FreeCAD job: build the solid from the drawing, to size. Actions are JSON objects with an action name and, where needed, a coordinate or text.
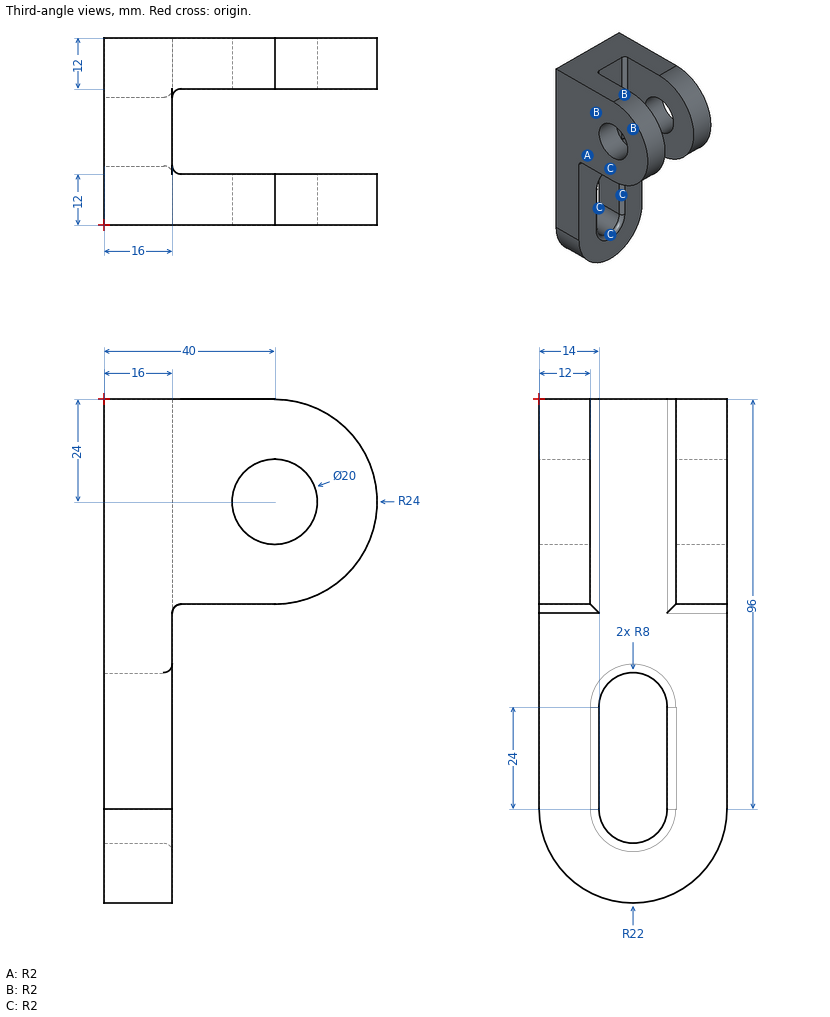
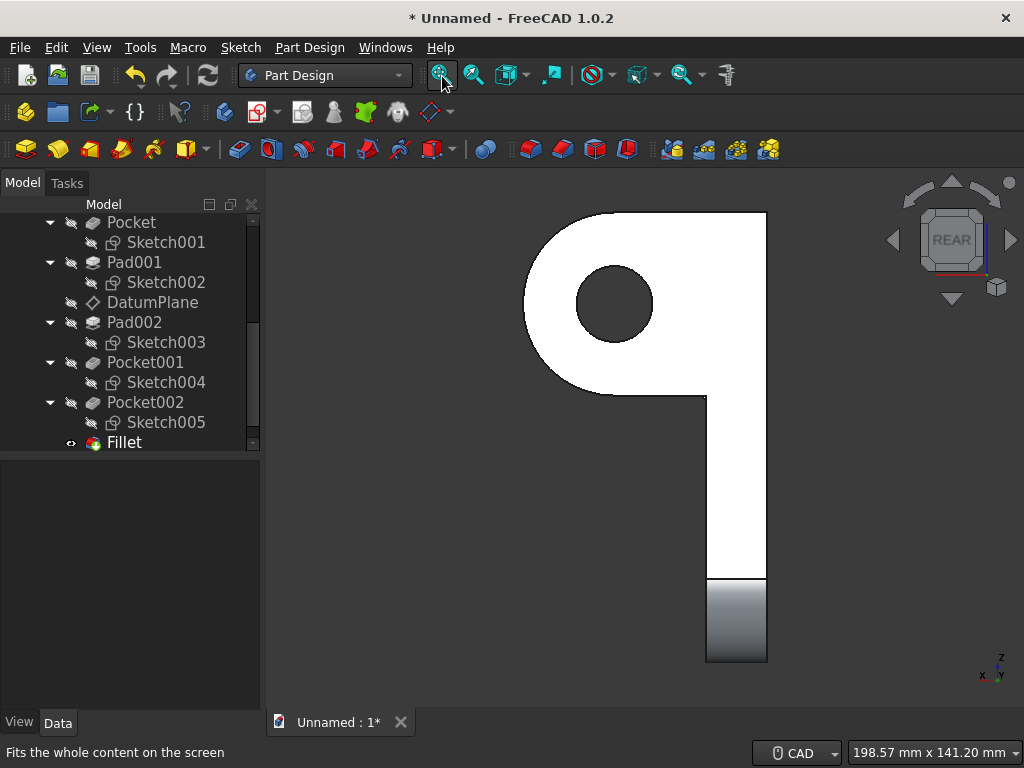
{"action": "key", "text": "6"}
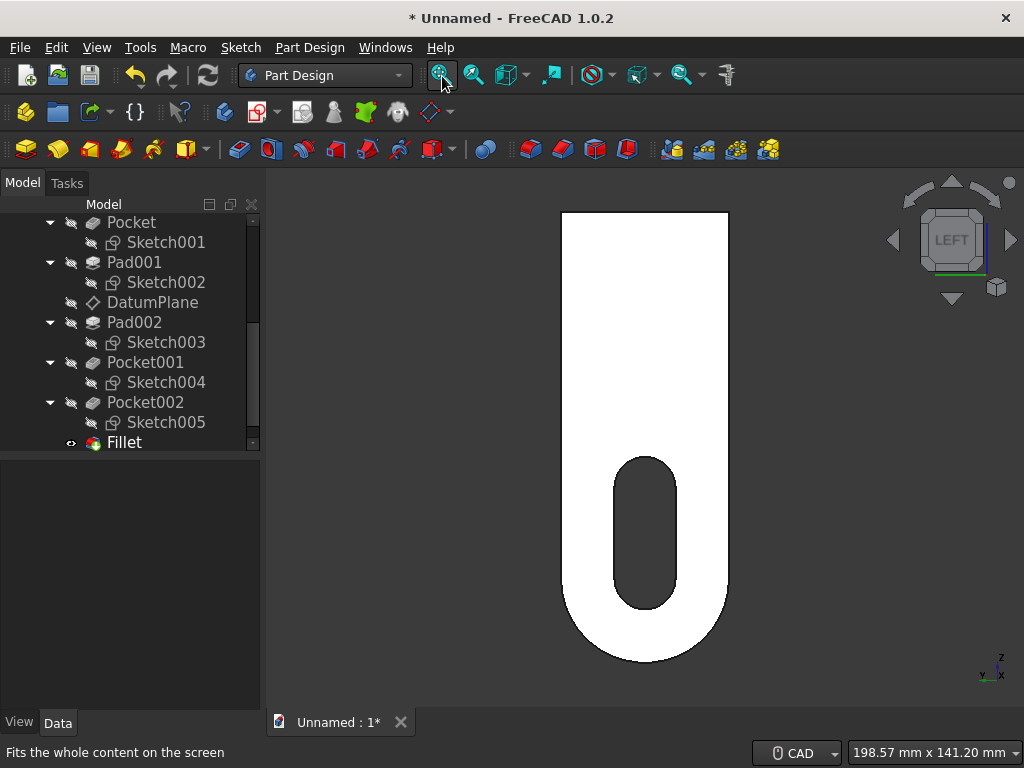
{"action": "key", "text": "v 3"}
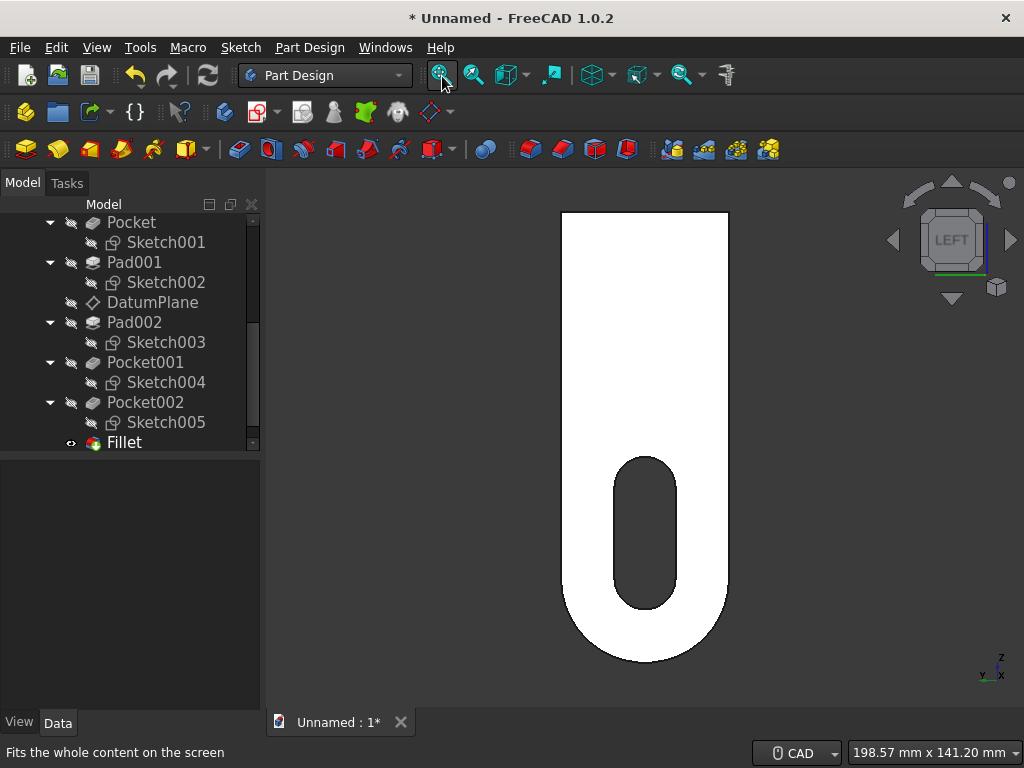
{"action": "key", "text": "0"}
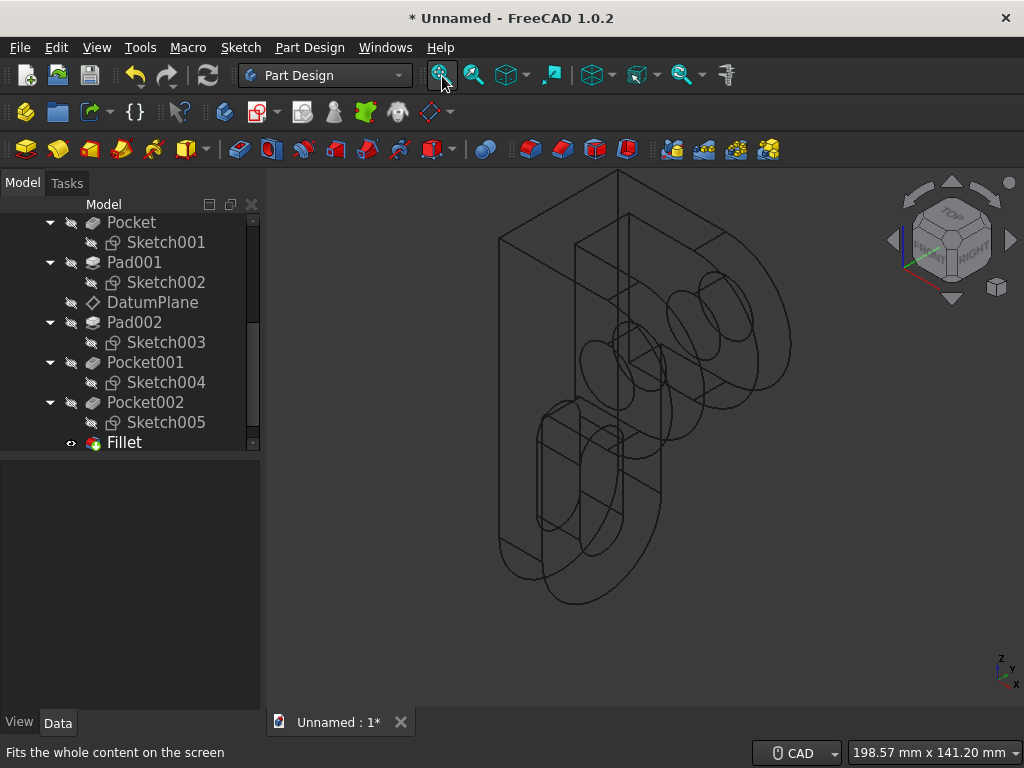
{"action": "left_click", "coordinate": [575, 318]}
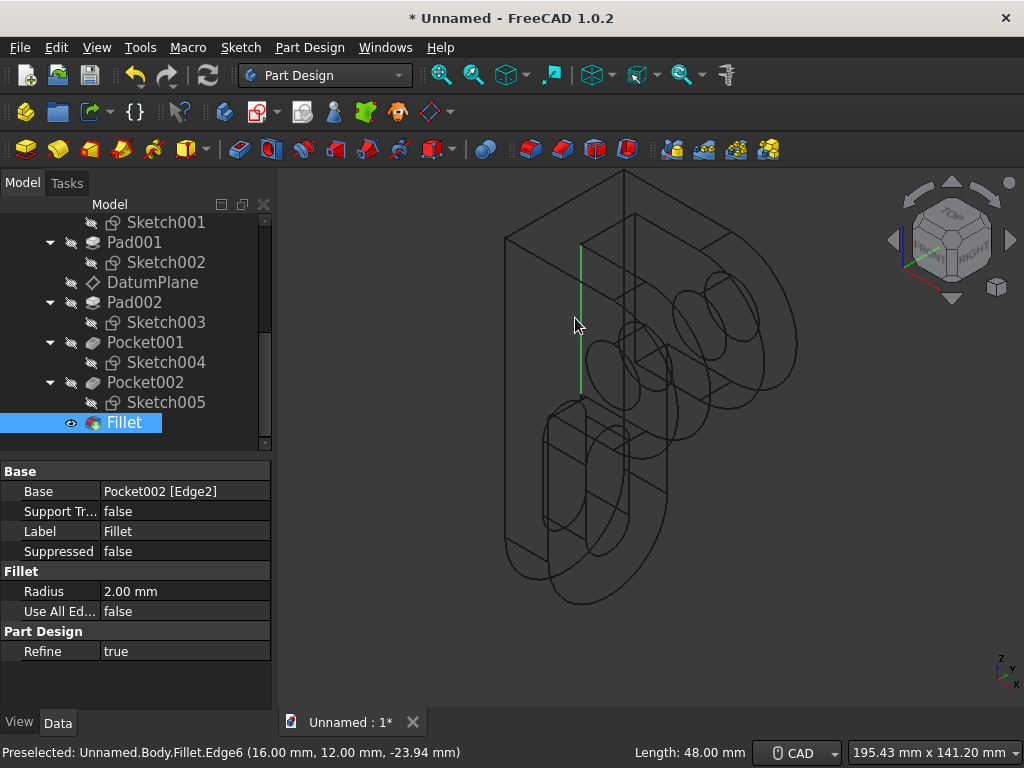
{"action": "left_click", "coordinate": [635, 302], "text": "ctrl"}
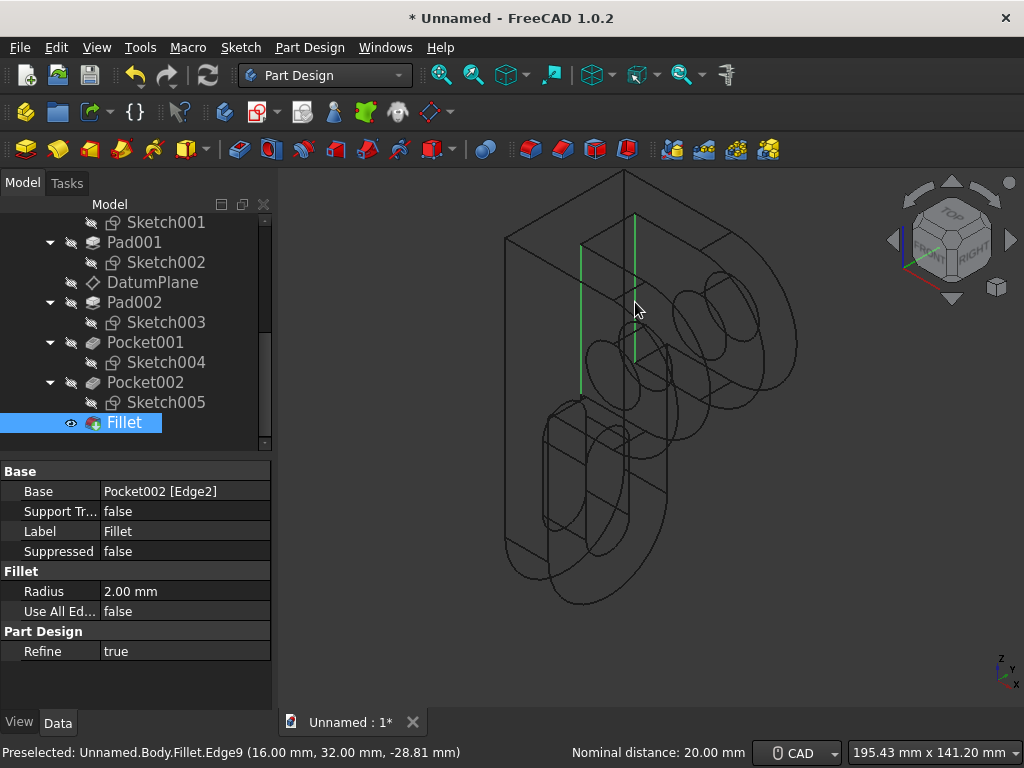
{"action": "left_click", "coordinate": [651, 352], "text": "ctrl"}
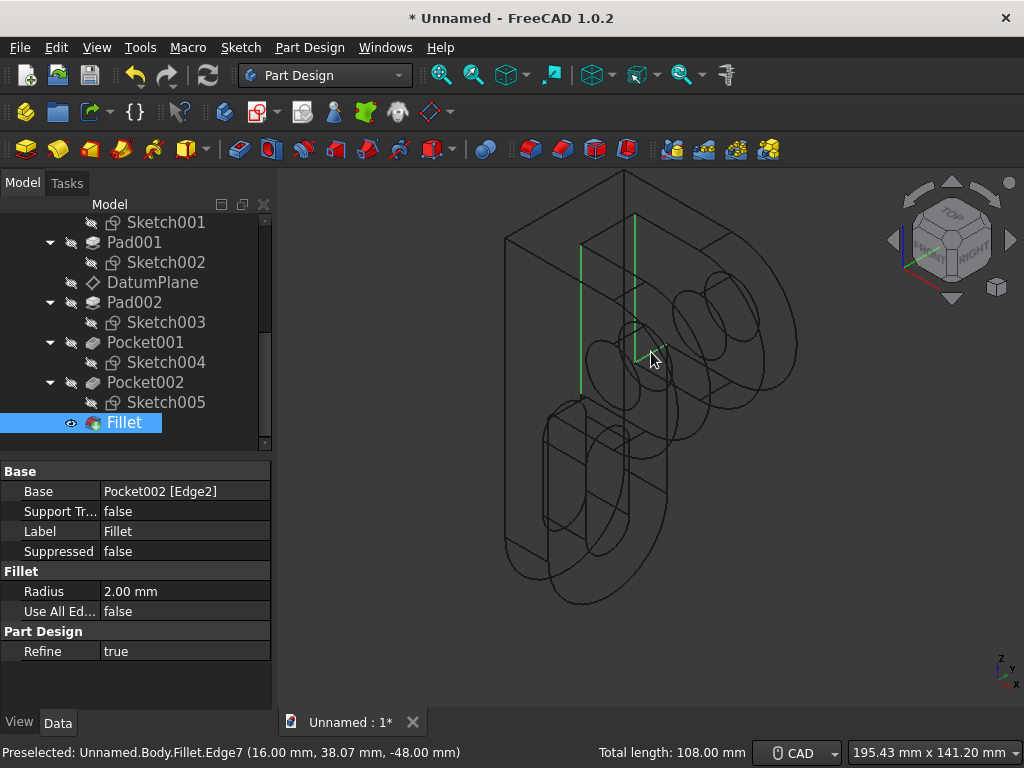
{"action": "key", "text": "v 1"}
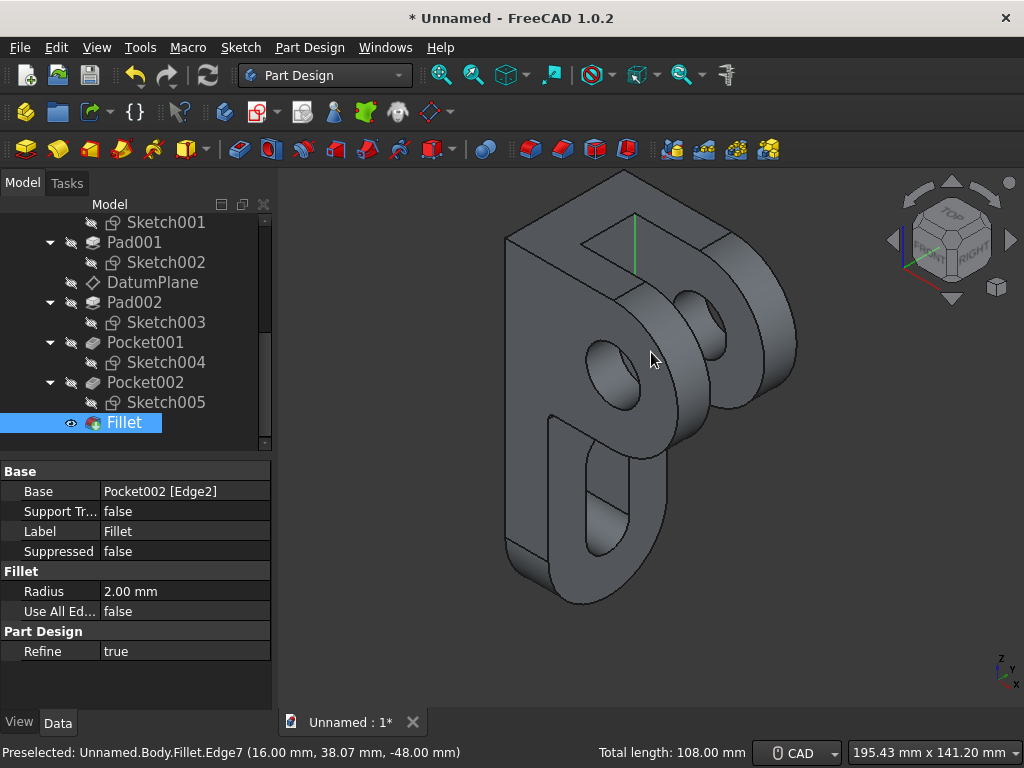
{"action": "left_click", "coordinate": [532, 150]}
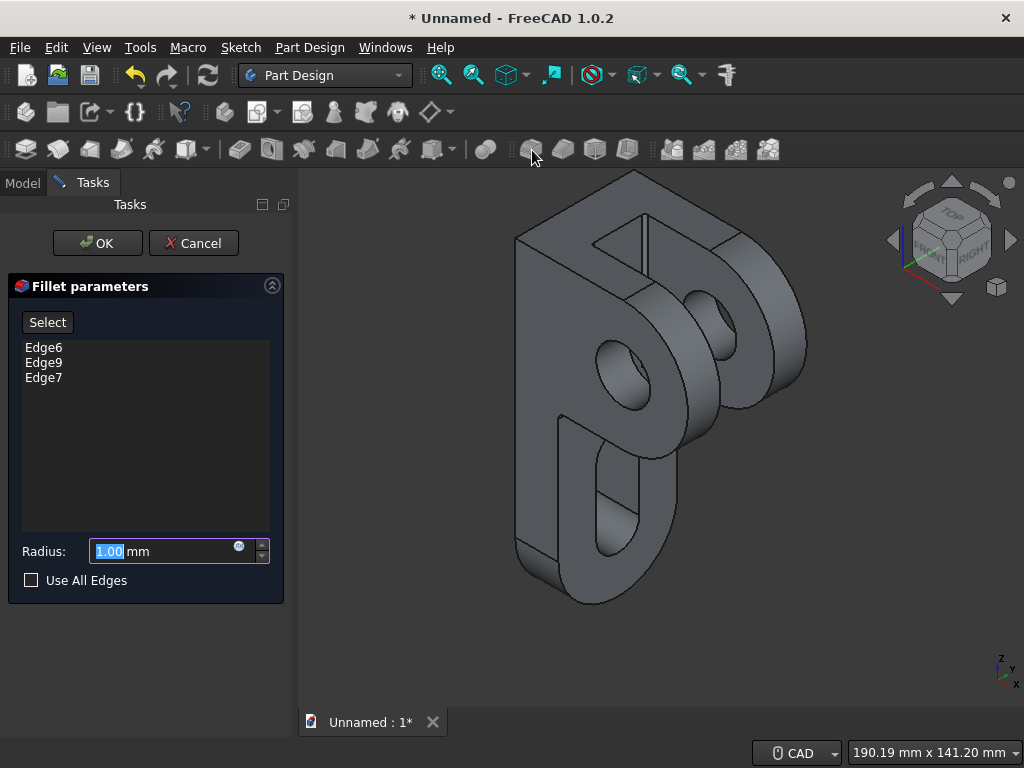
{"action": "type", "text": "2"}
{"action": "key", "text": "Tab"}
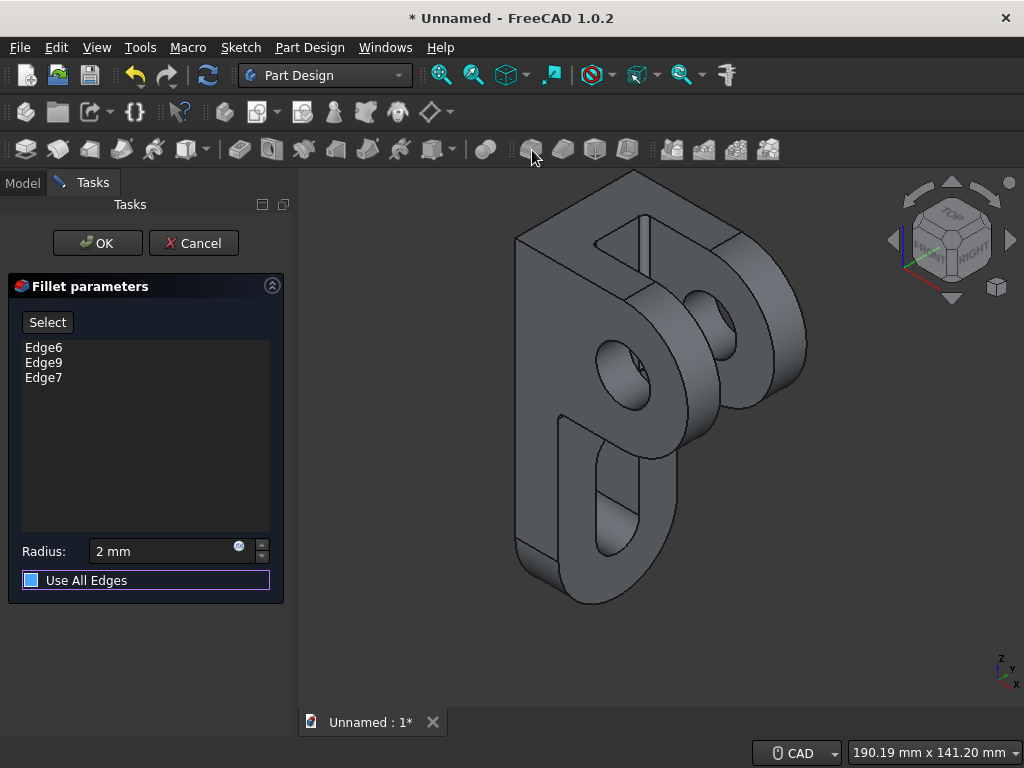
{"action": "left_click", "coordinate": [98, 243]}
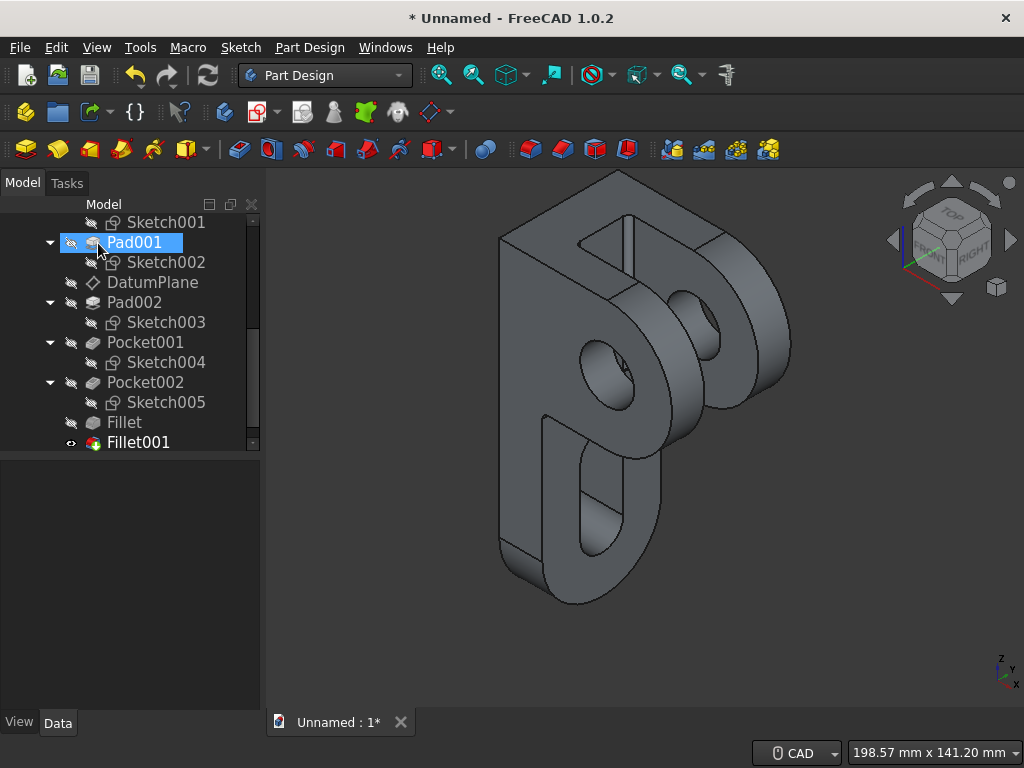
{"action": "left_click", "coordinate": [602, 552]}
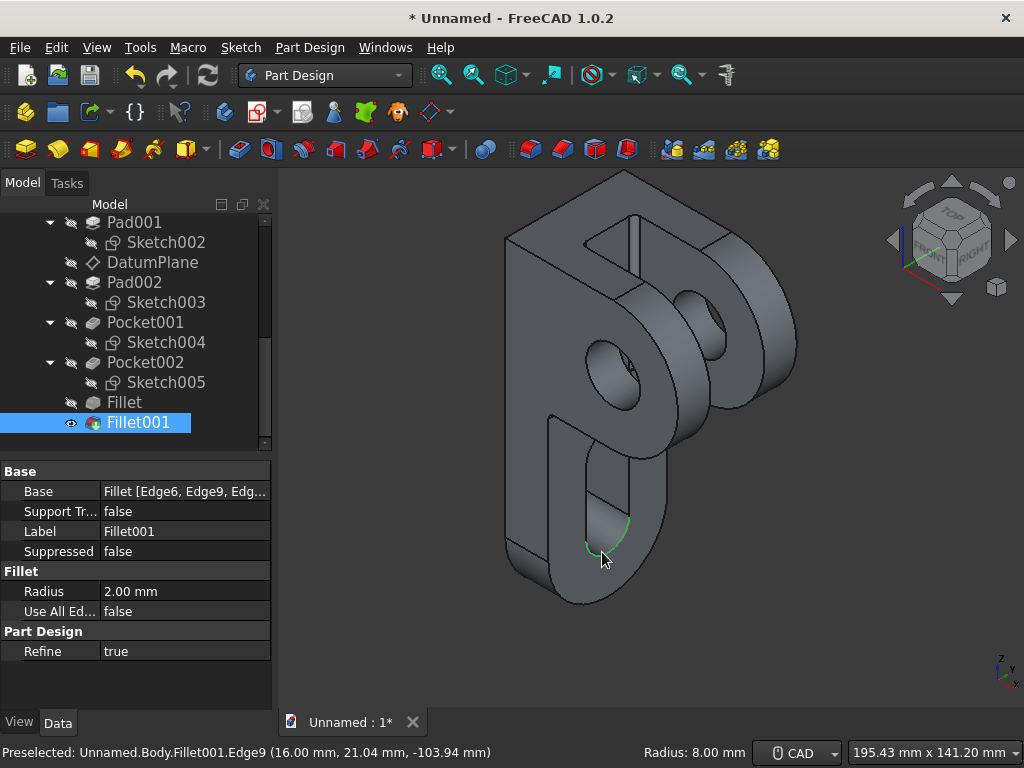
{"action": "left_click", "coordinate": [629, 477], "text": "ctrl"}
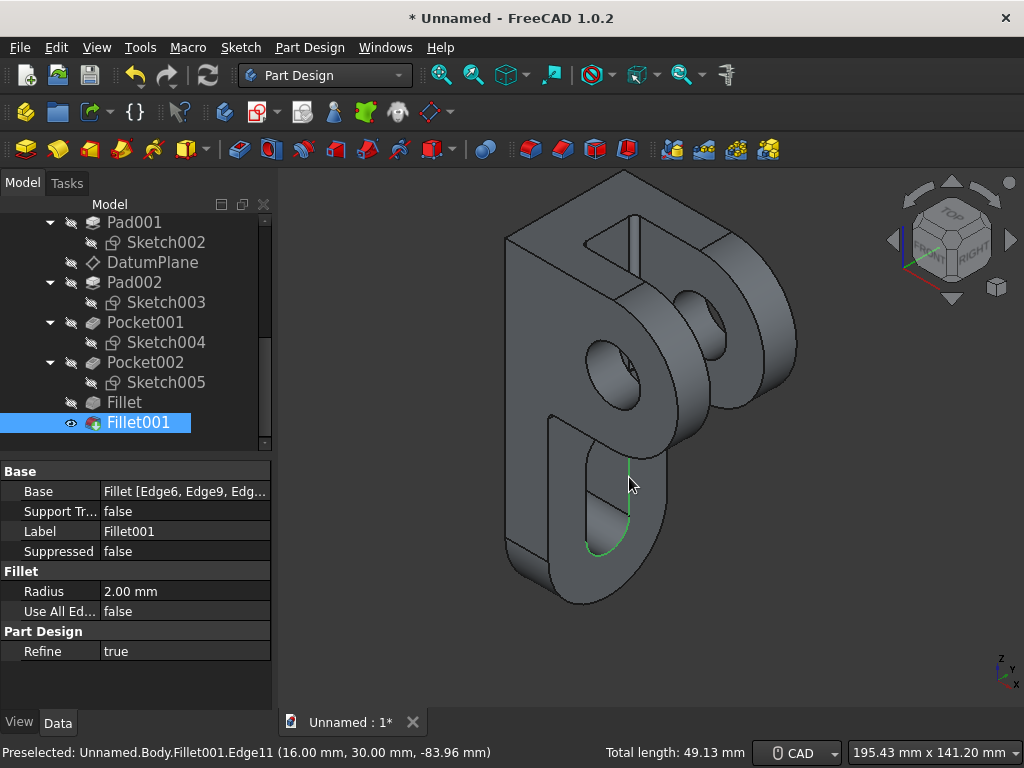
{"action": "key", "text": "2"}